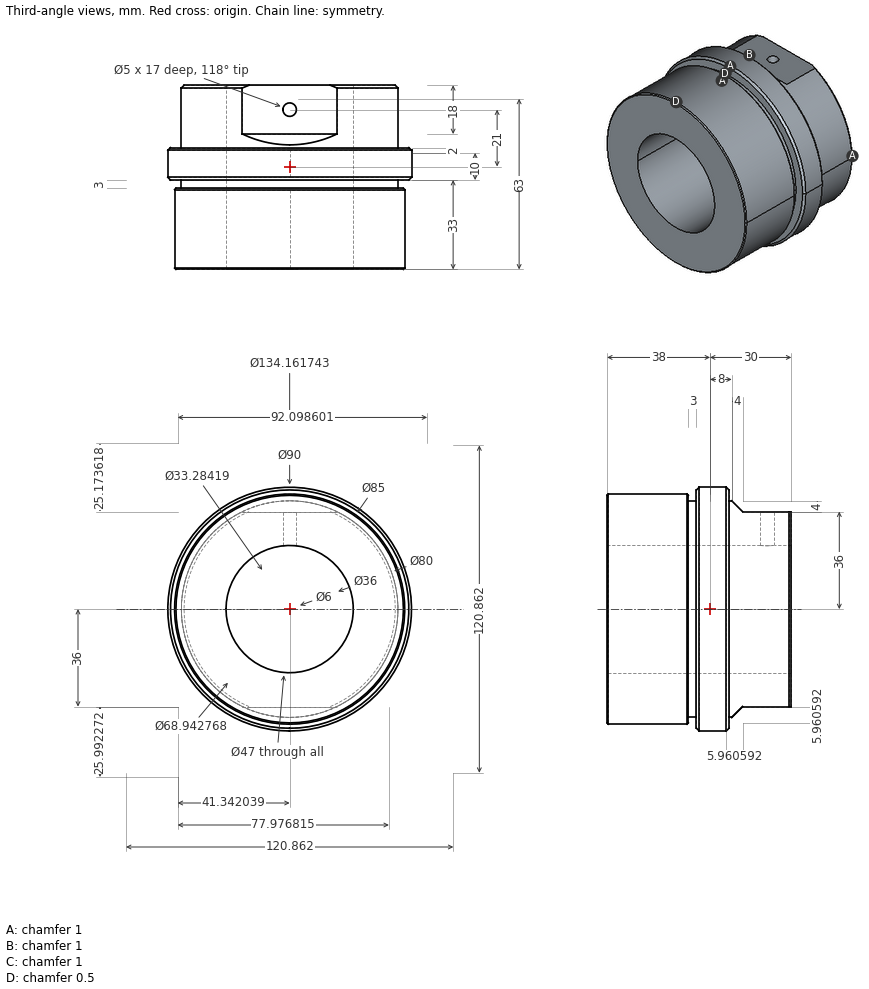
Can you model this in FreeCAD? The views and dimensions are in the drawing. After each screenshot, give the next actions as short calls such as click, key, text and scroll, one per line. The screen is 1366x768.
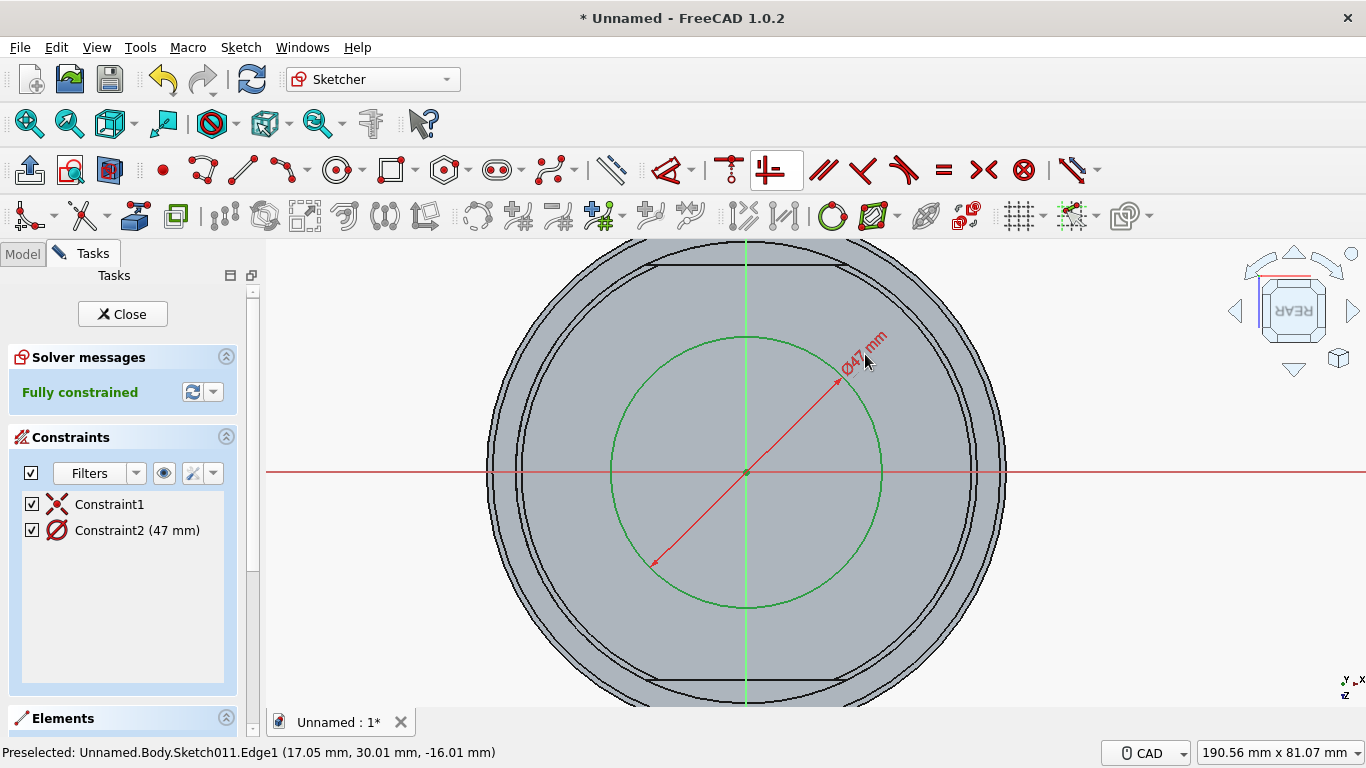
click(123, 314)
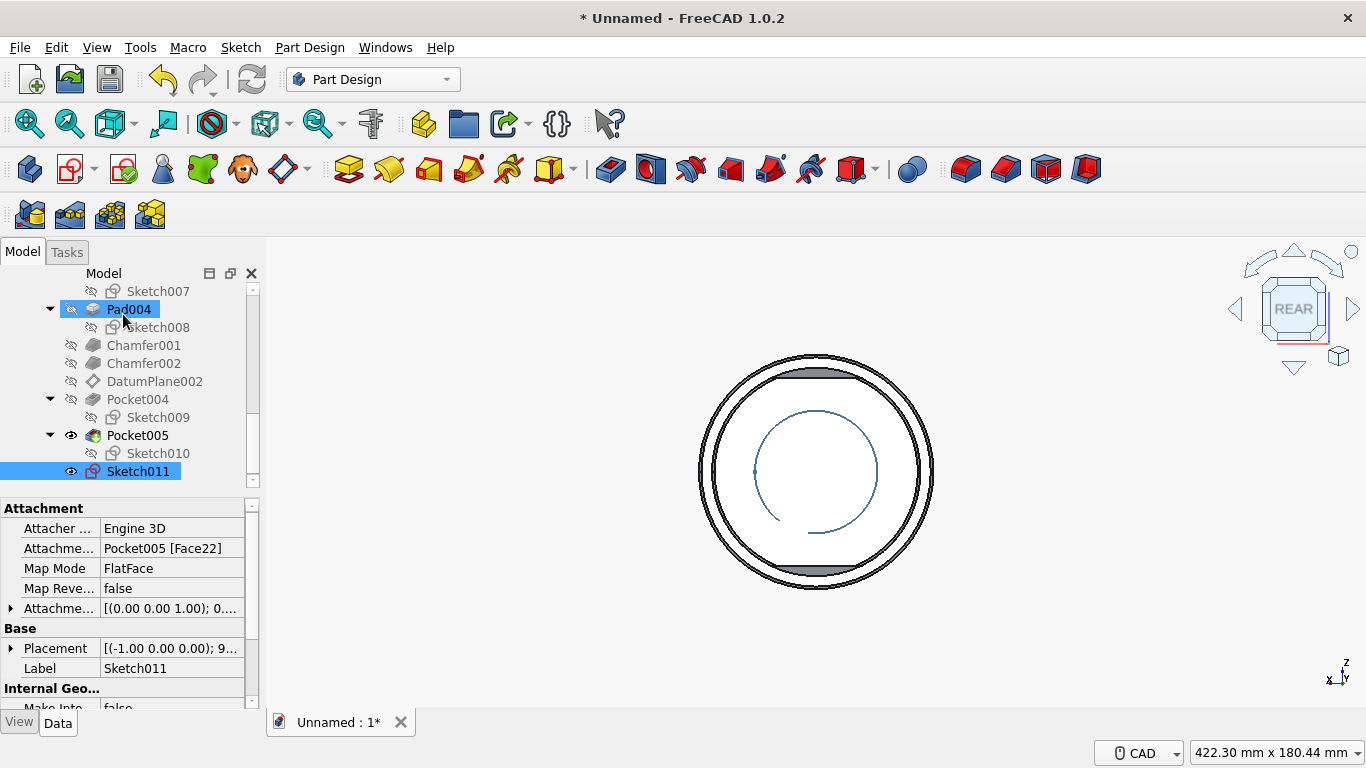
click(652, 170)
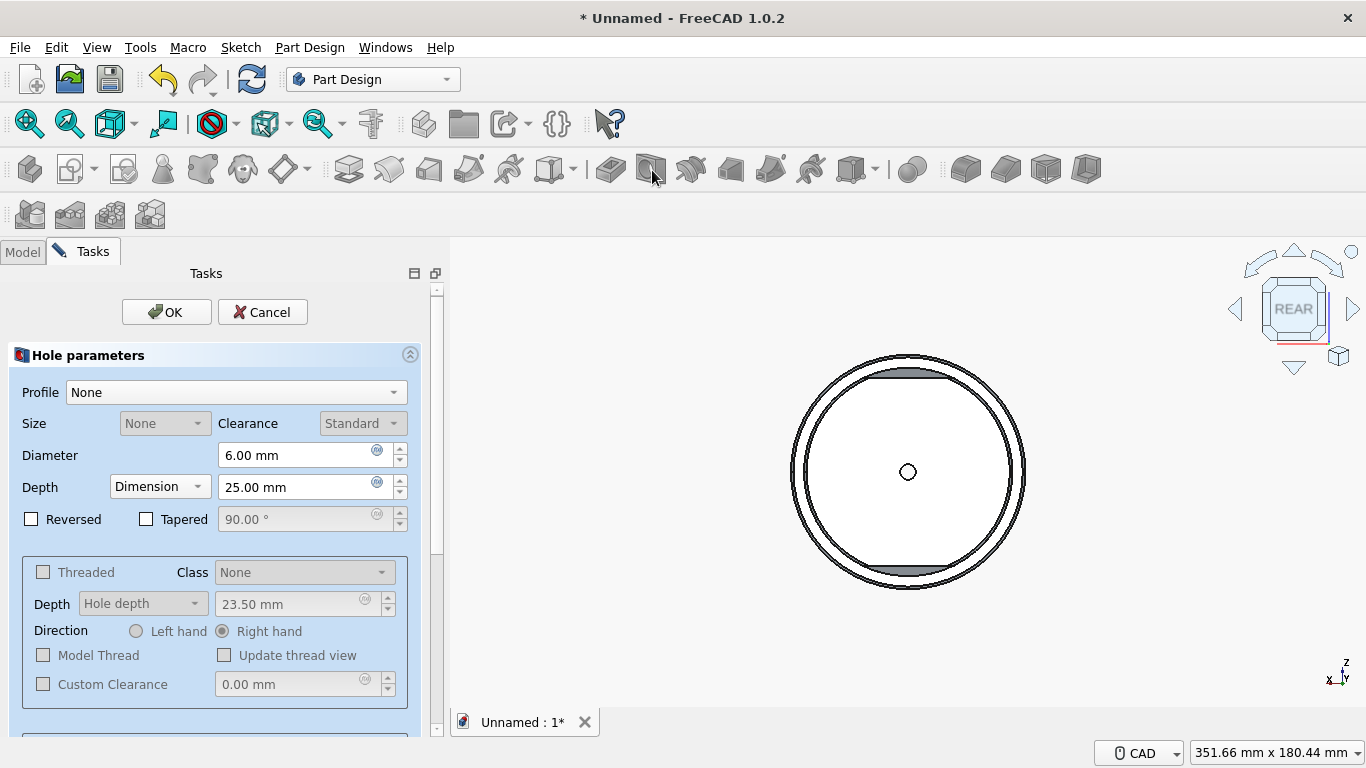
triple_click(305, 455)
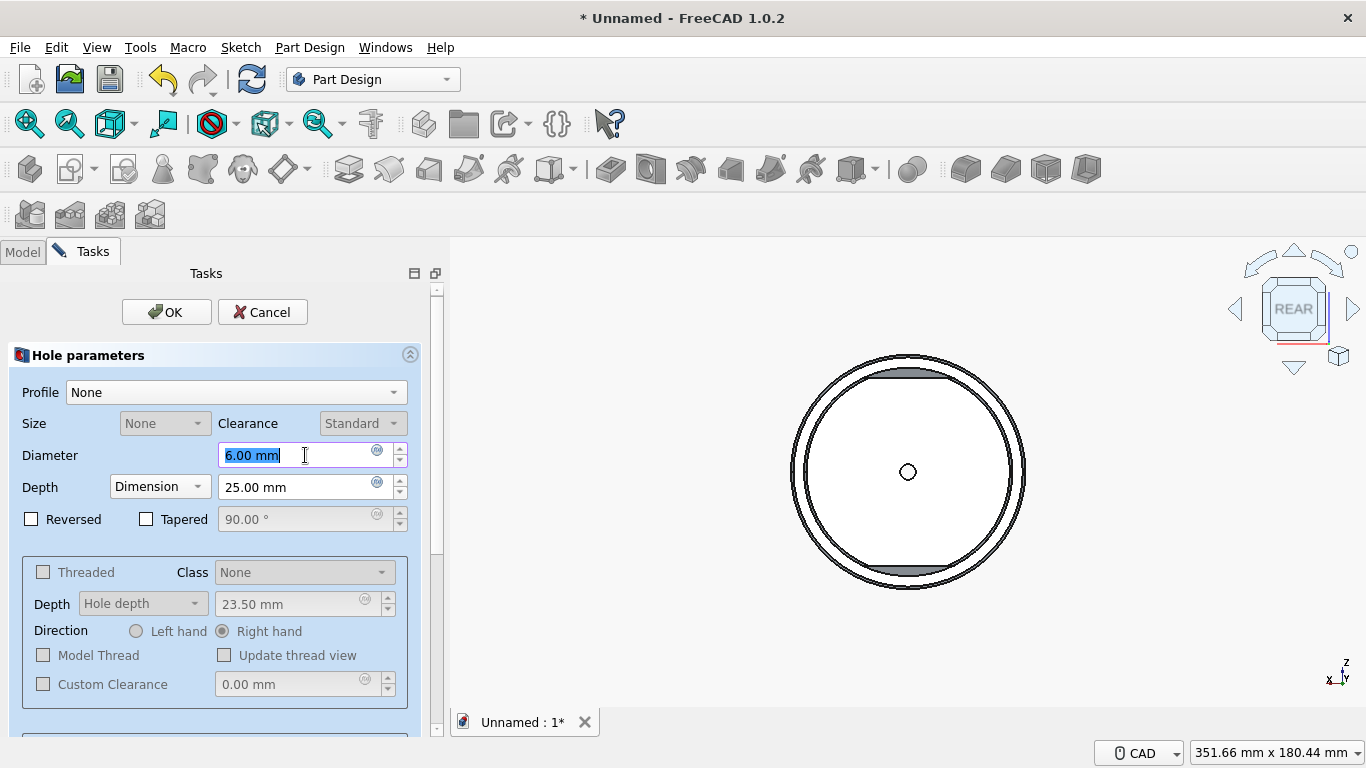
text(47)
key(Tab)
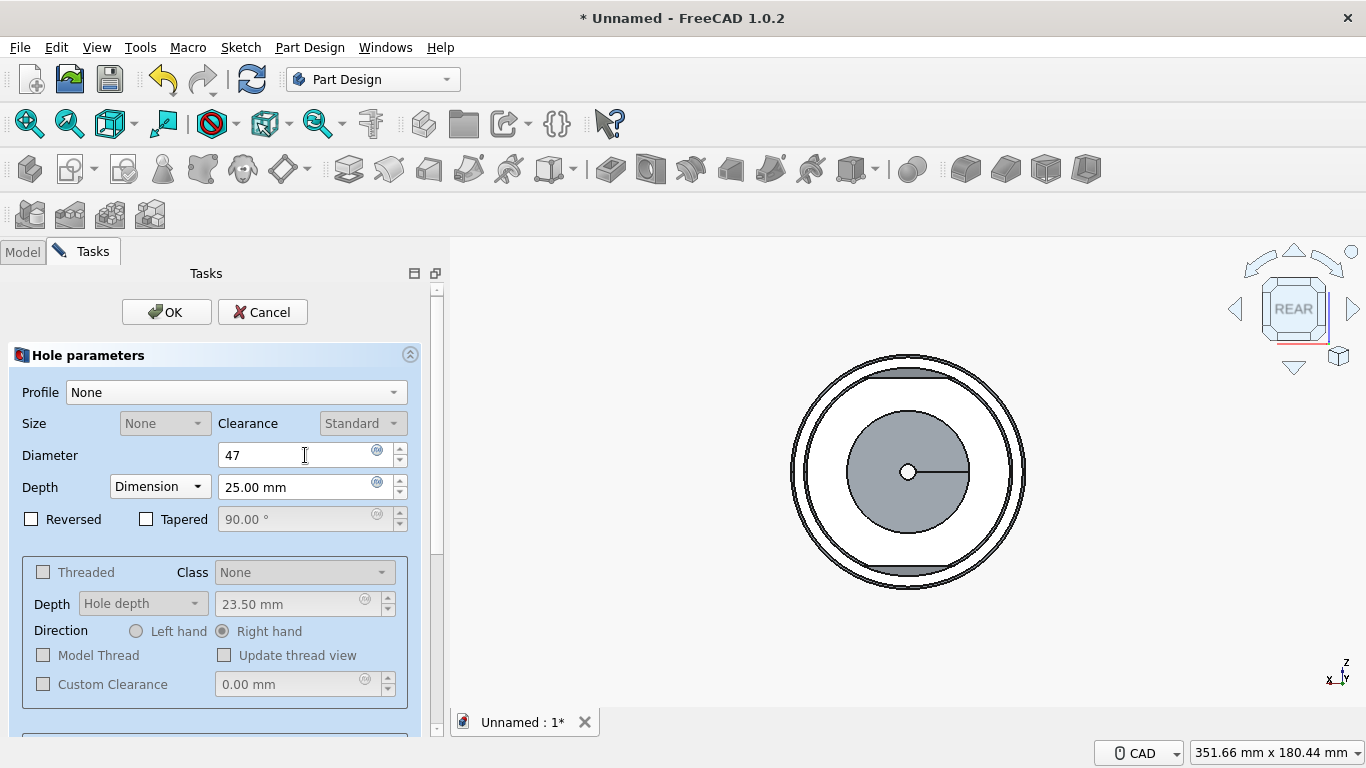
click(161, 486)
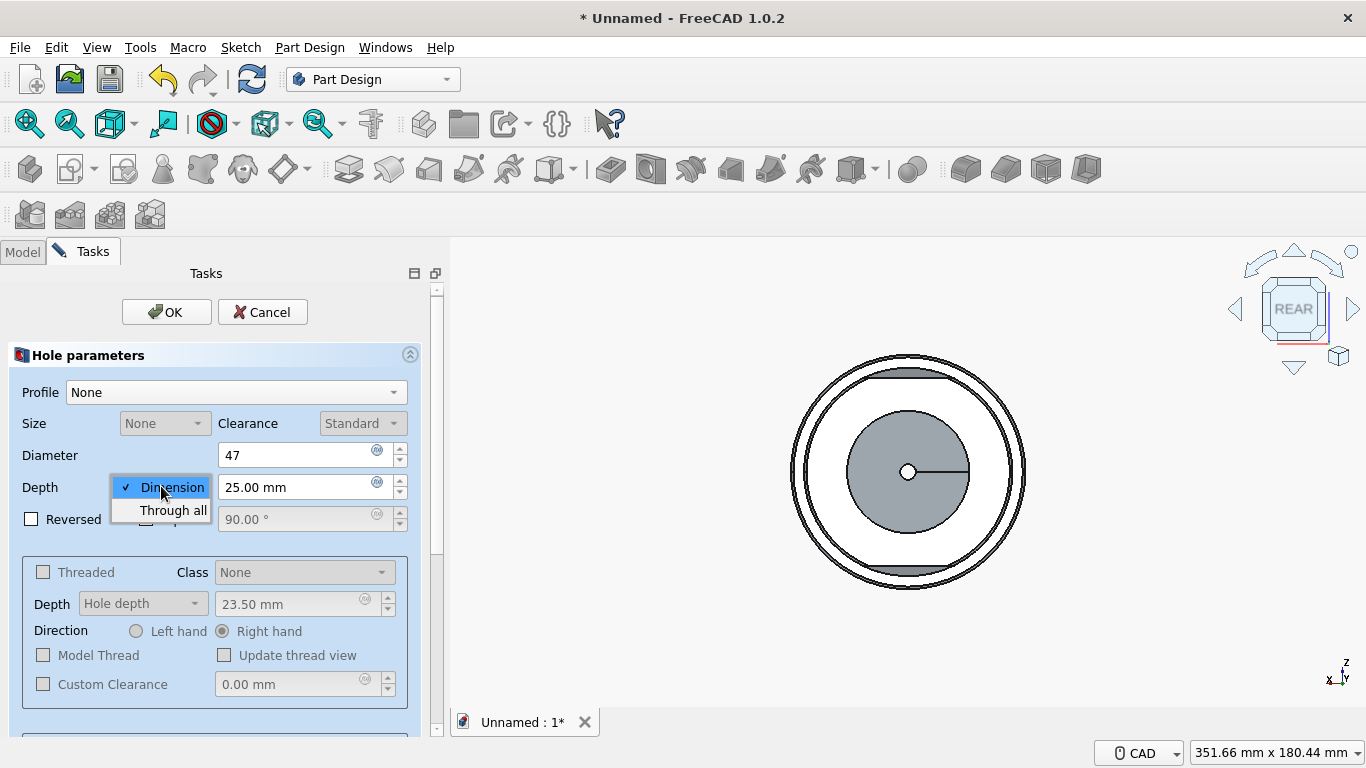
click(160, 510)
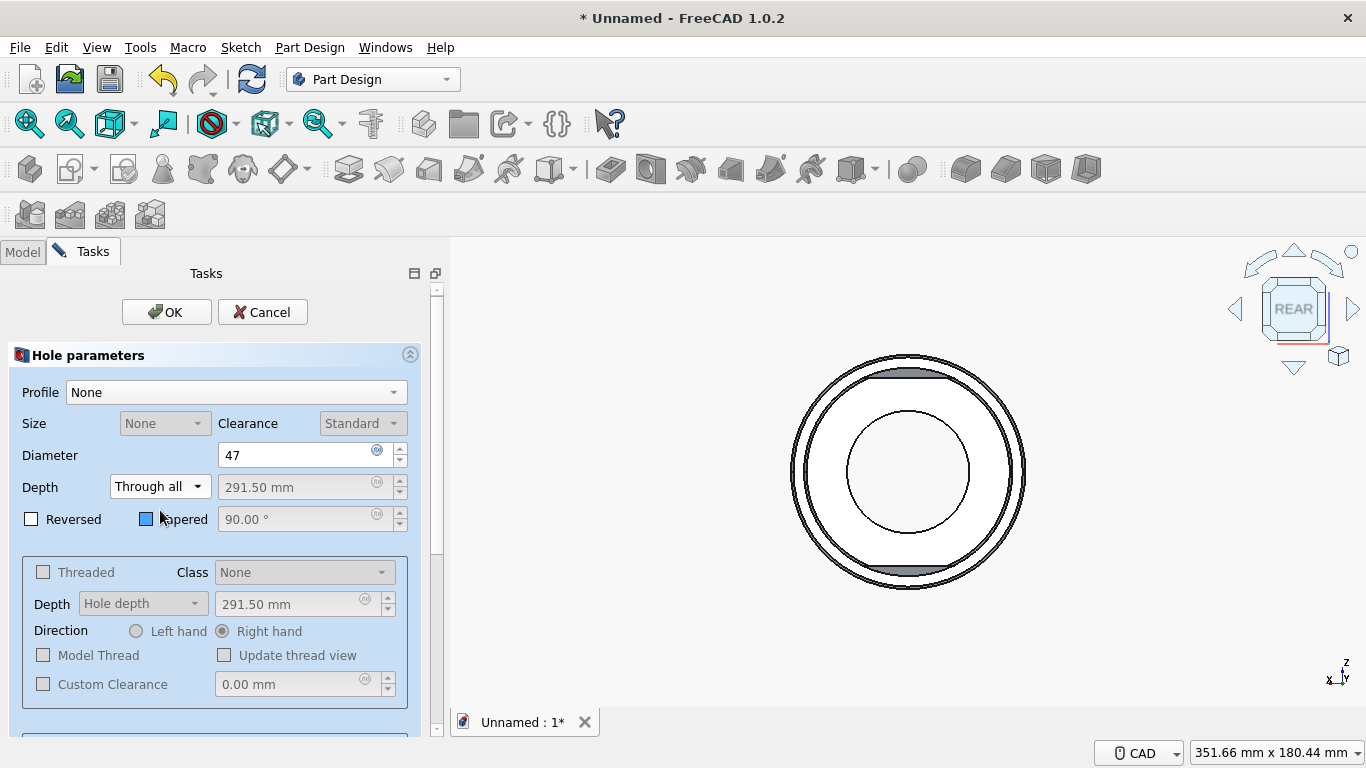
click(167, 312)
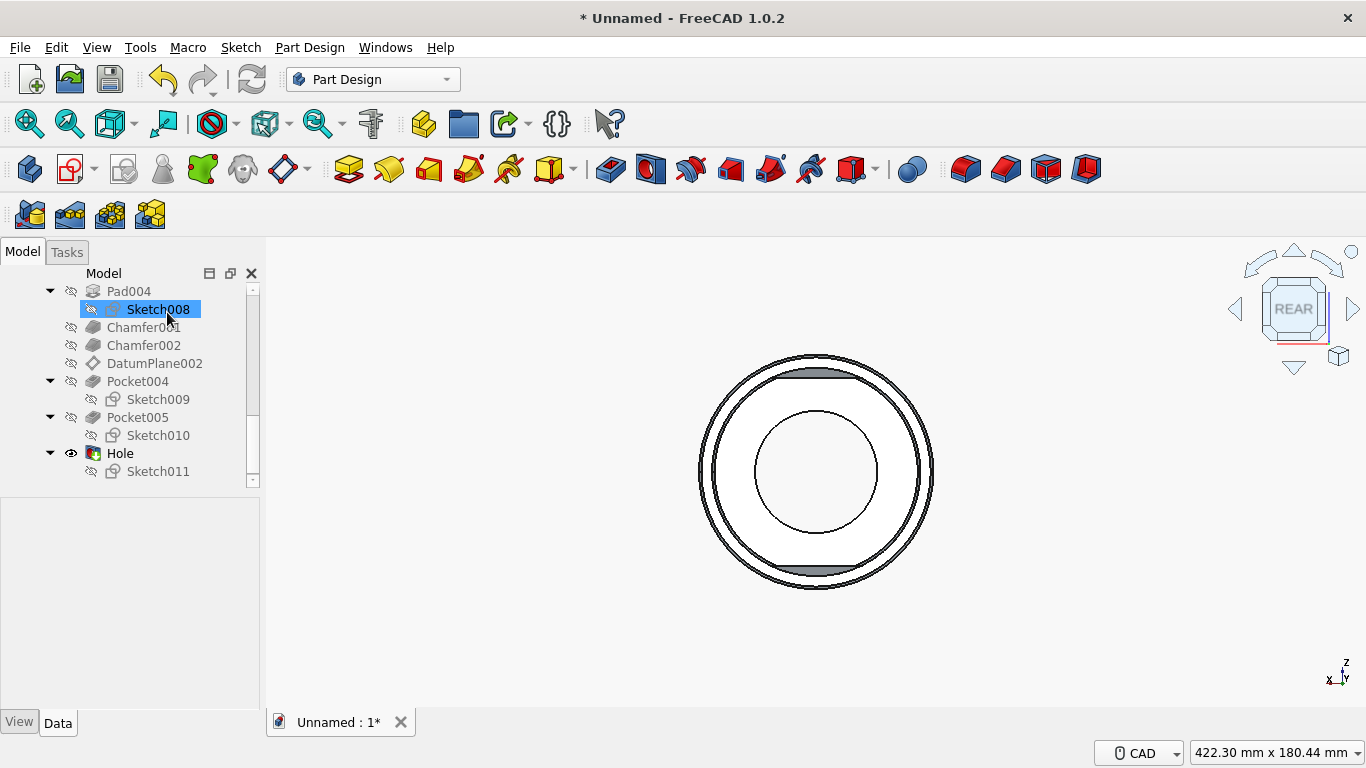
key(0)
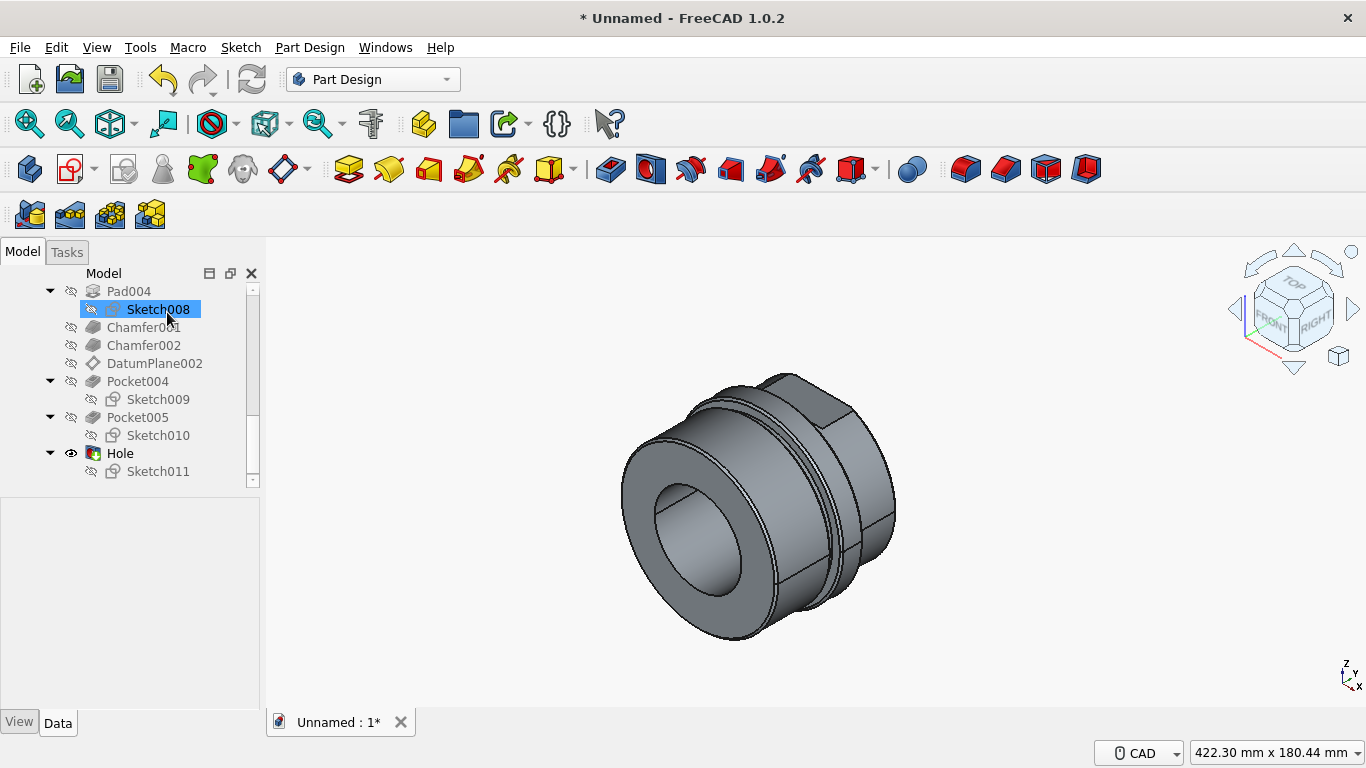
scroll(825, 494, up, 7)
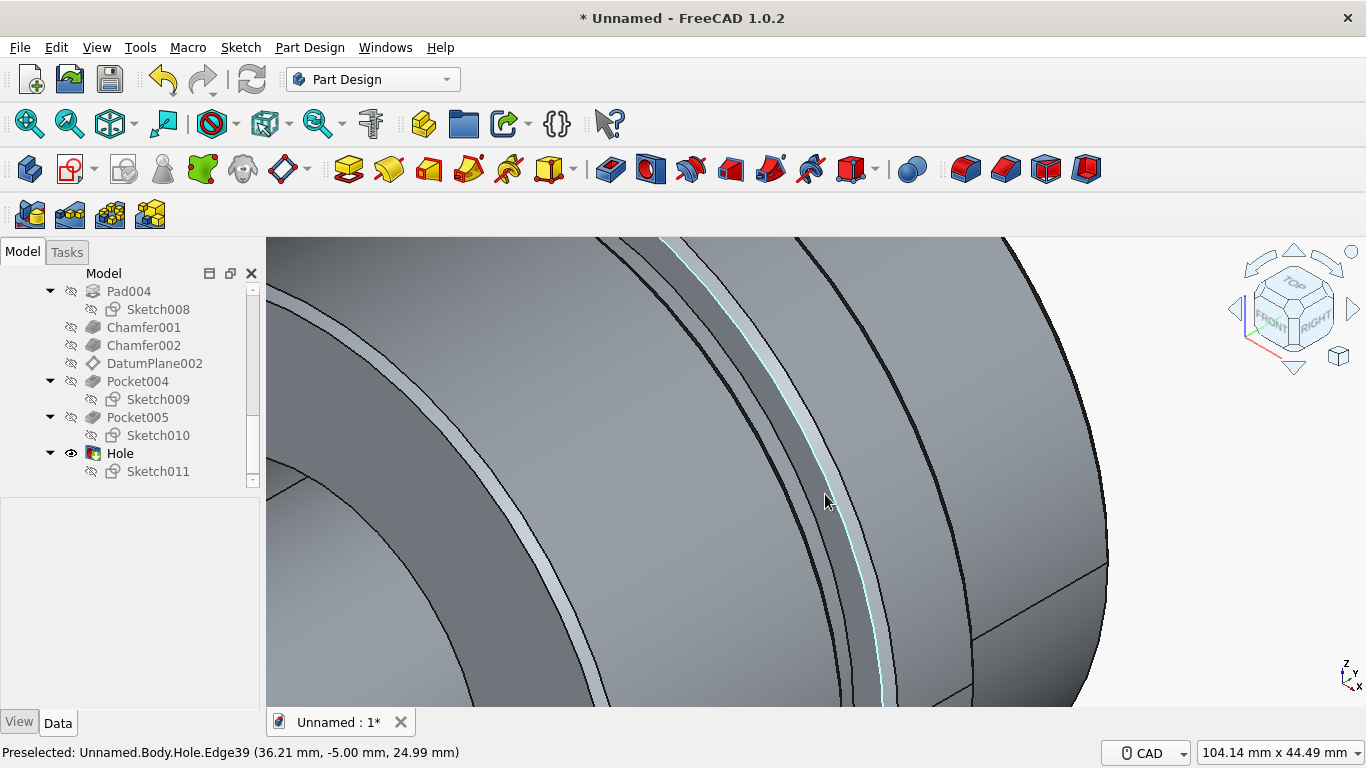
click(871, 669)